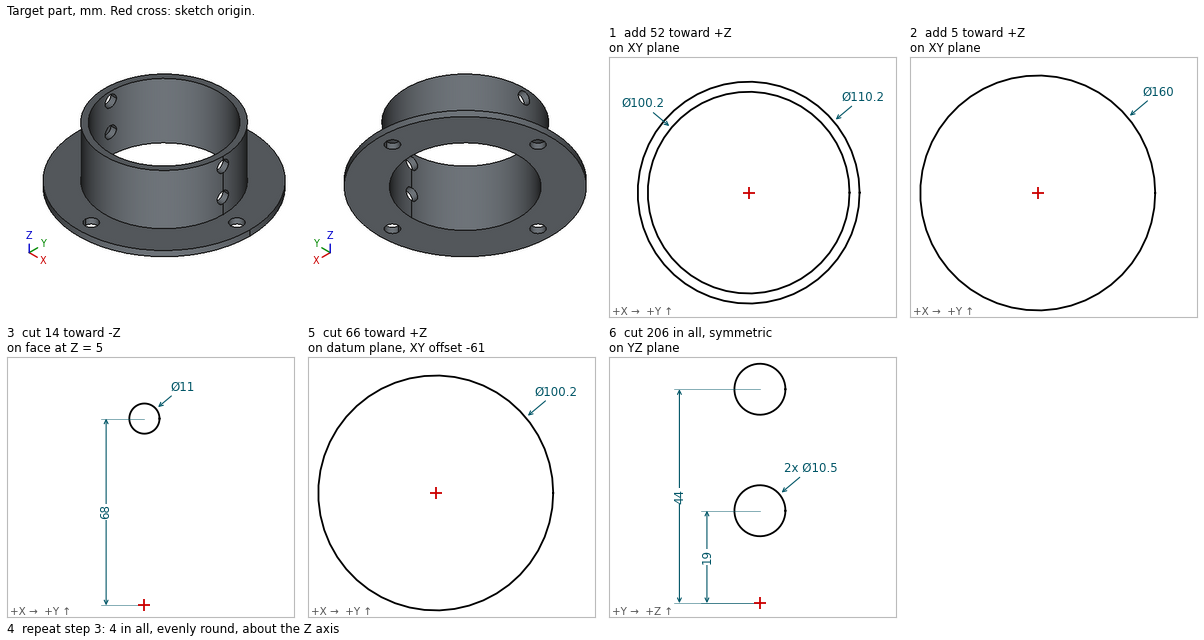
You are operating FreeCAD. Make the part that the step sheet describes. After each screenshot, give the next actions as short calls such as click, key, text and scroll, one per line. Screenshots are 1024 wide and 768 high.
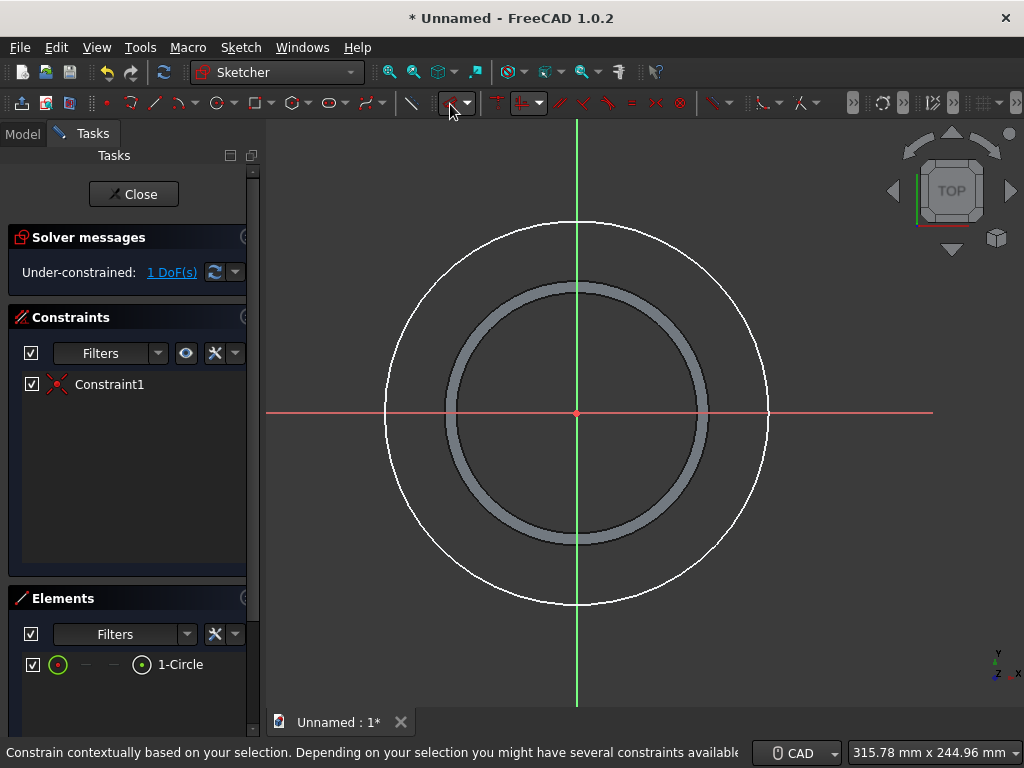
click(712, 277)
click(735, 254)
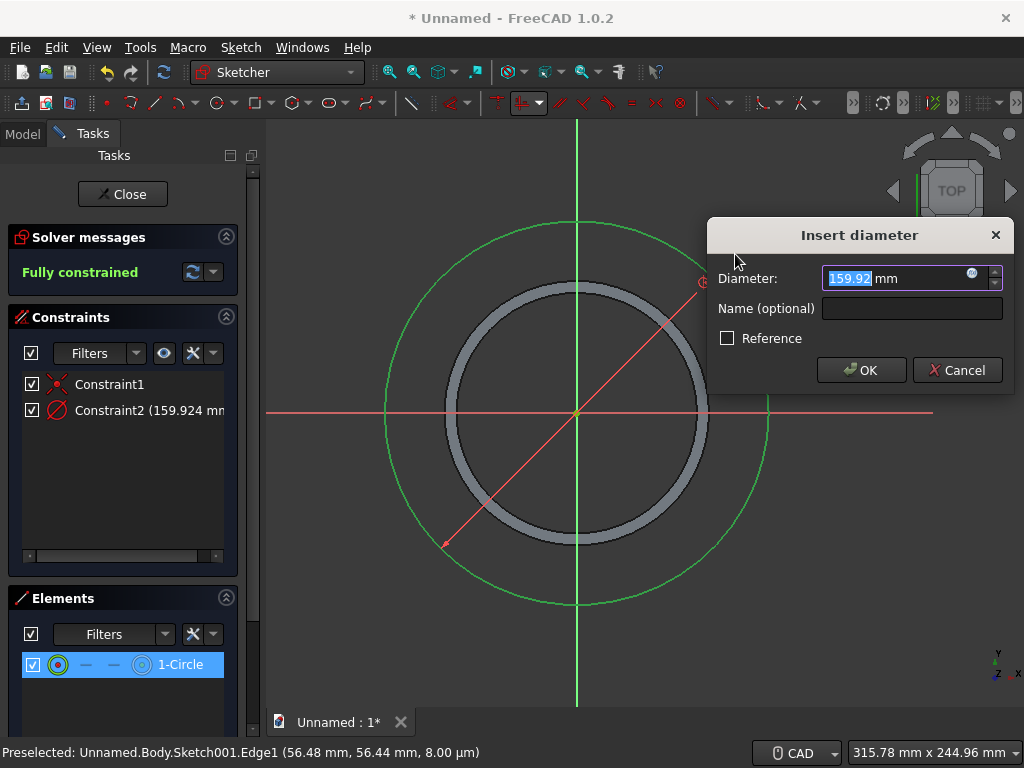
text(160)
key(Return)
key(Escape)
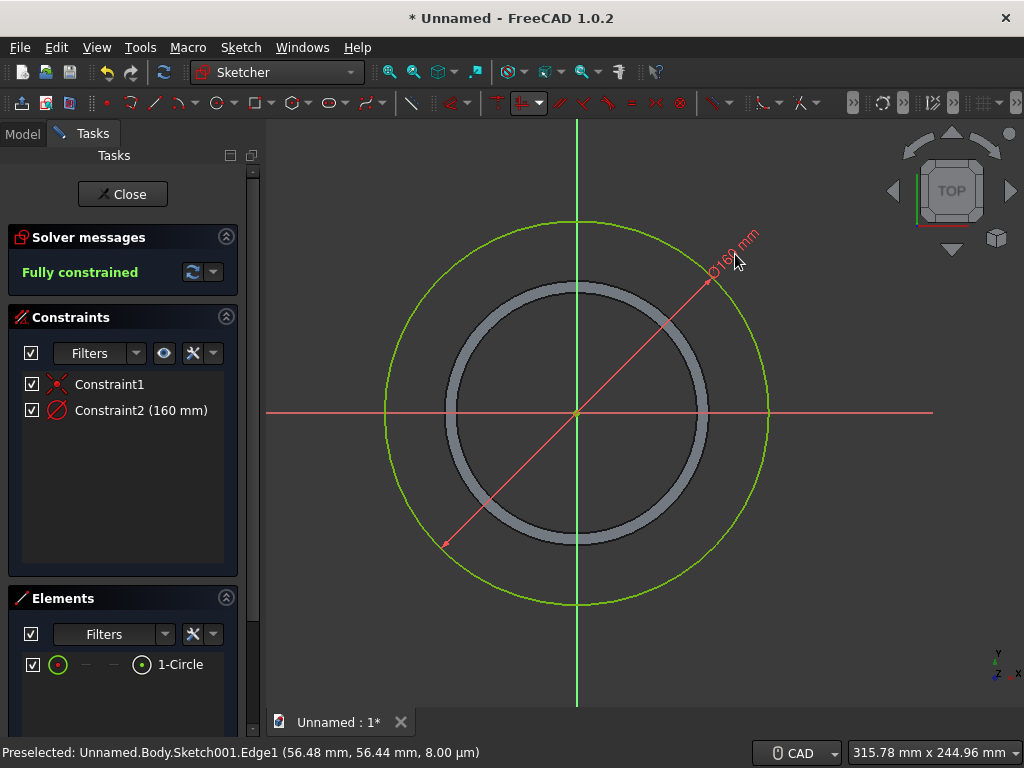
click(123, 194)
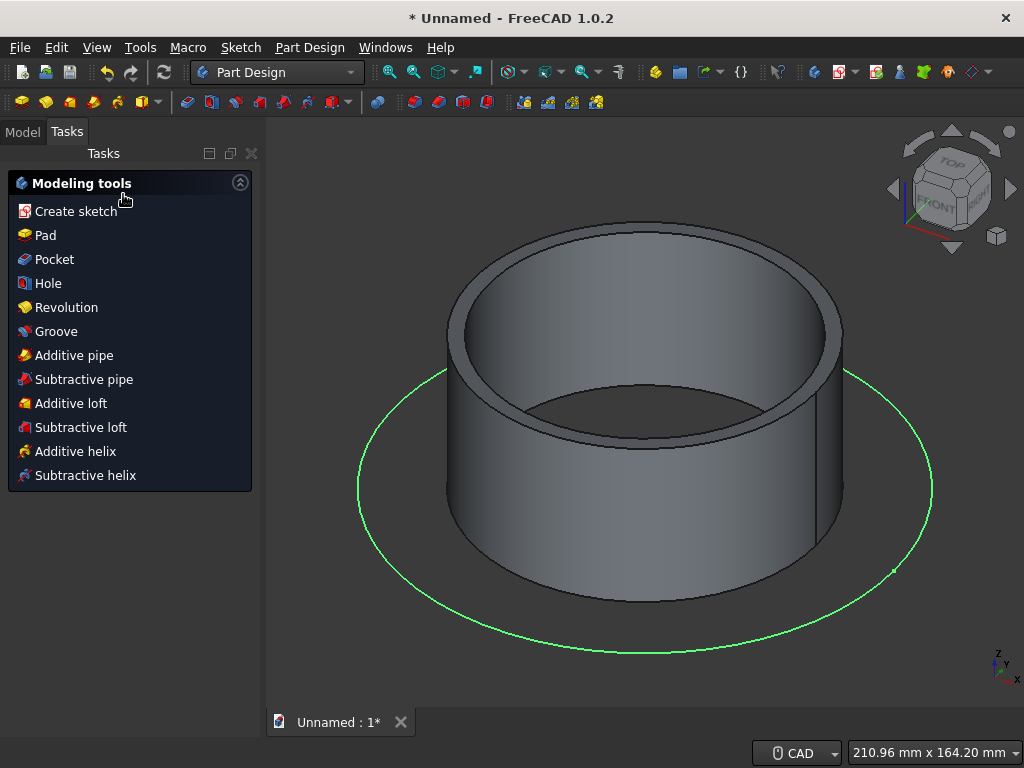
click(22, 102)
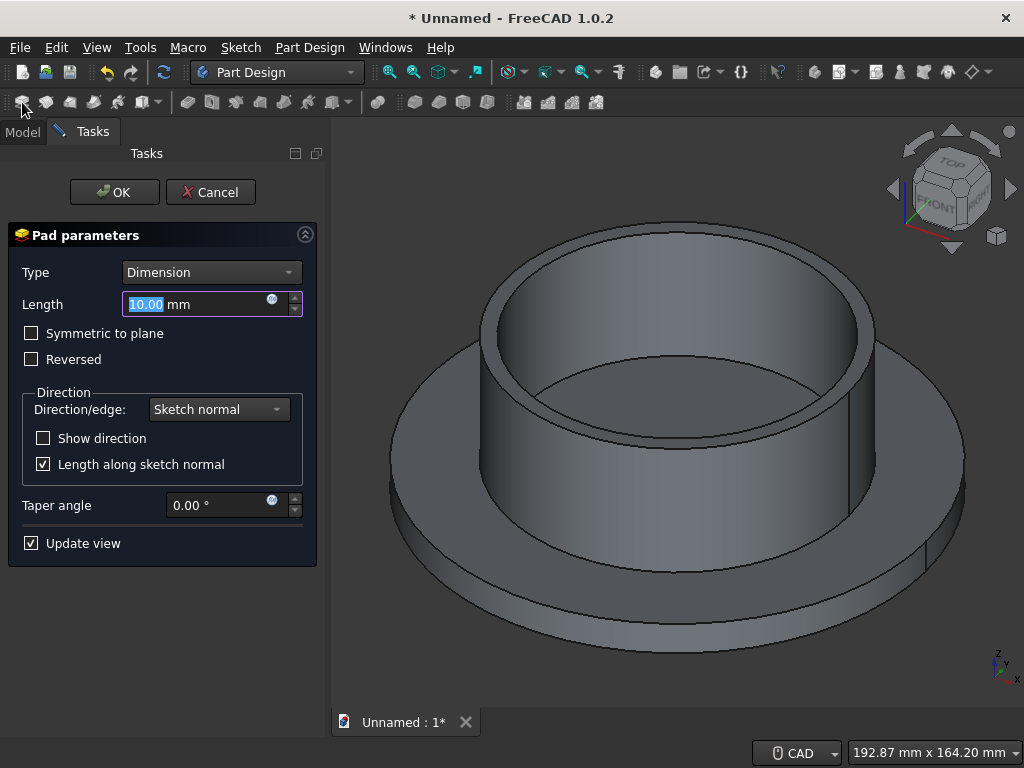
text(5)
key(Tab)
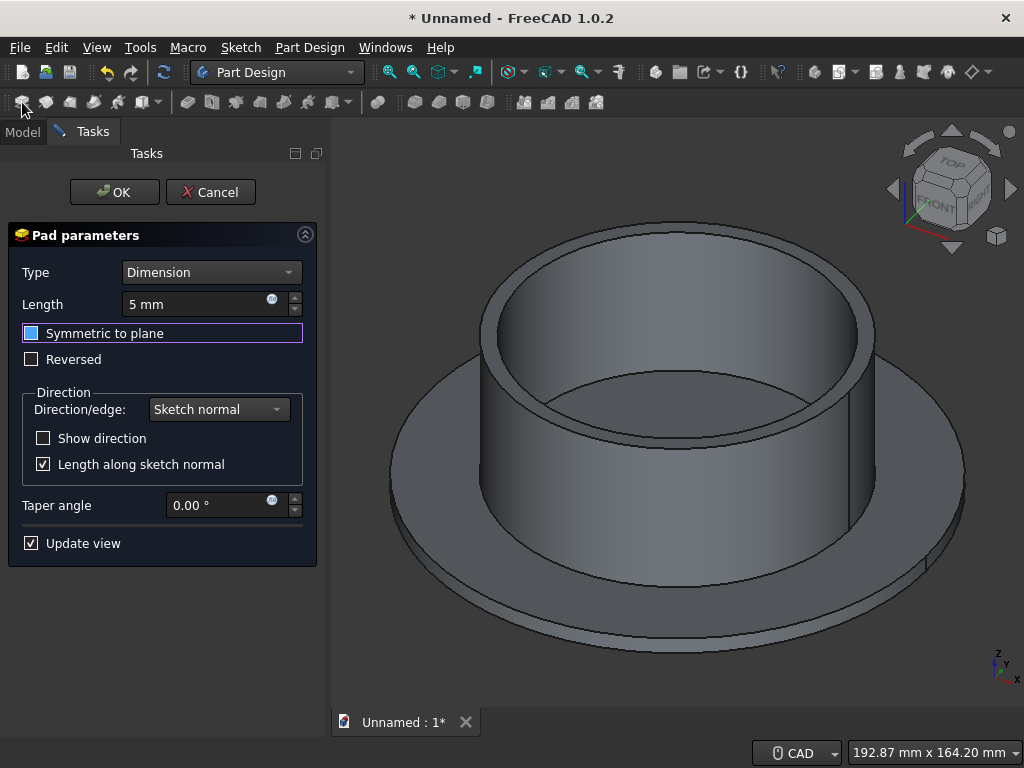
click(115, 192)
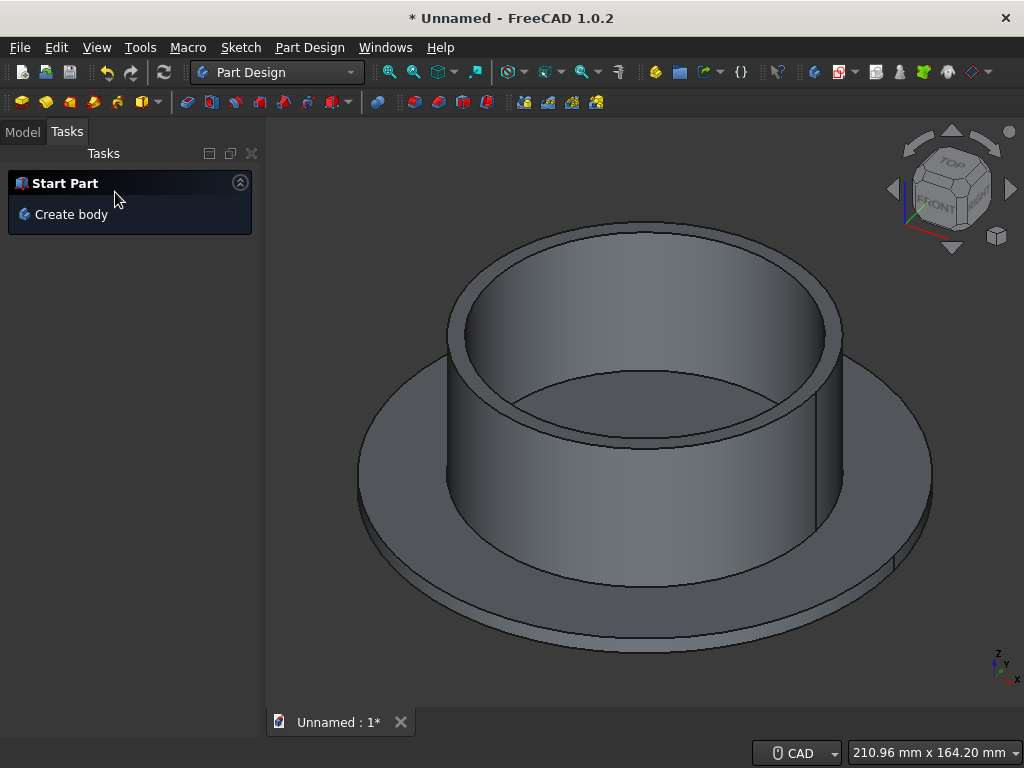
click(390, 72)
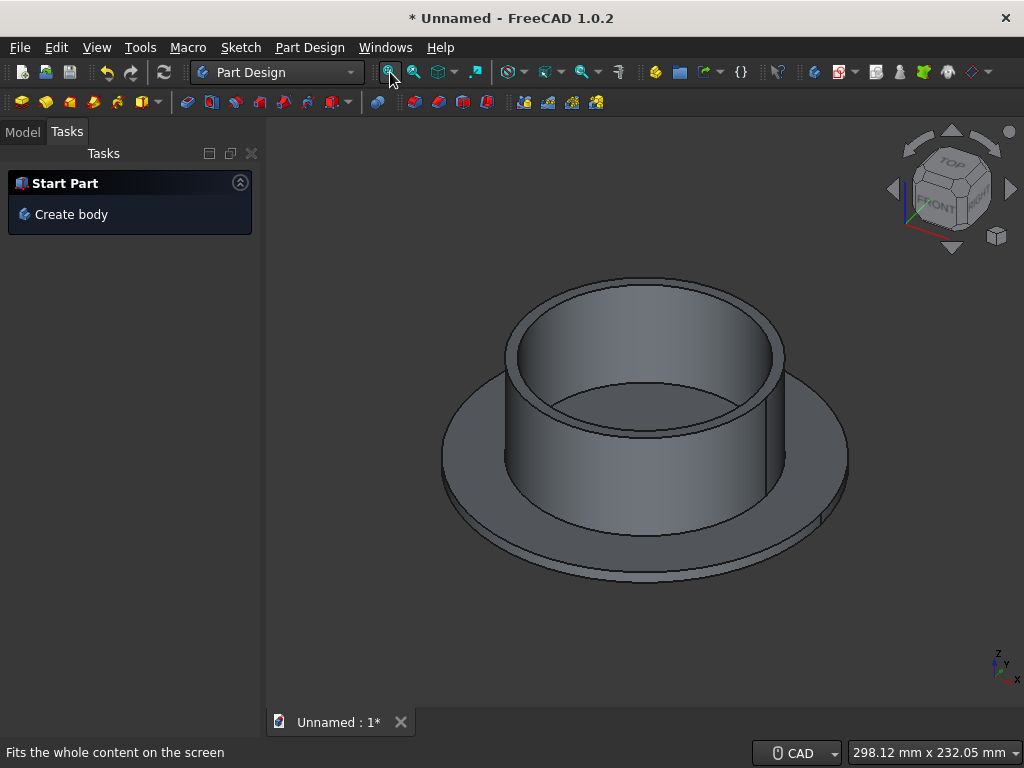
click(558, 541)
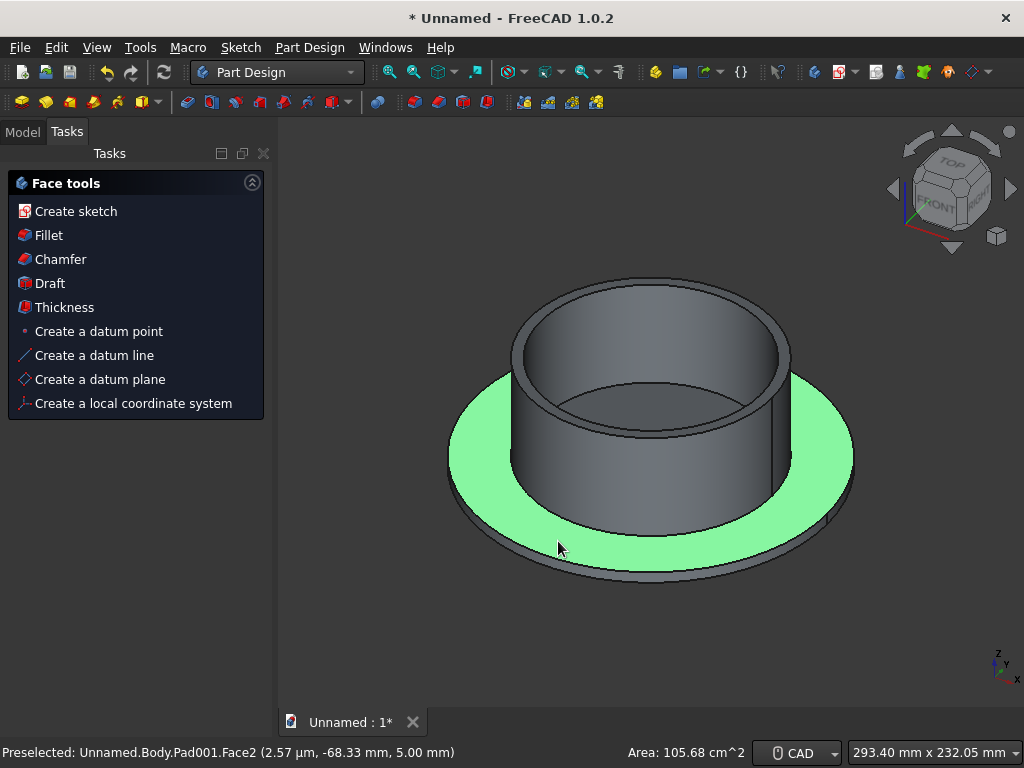
click(840, 72)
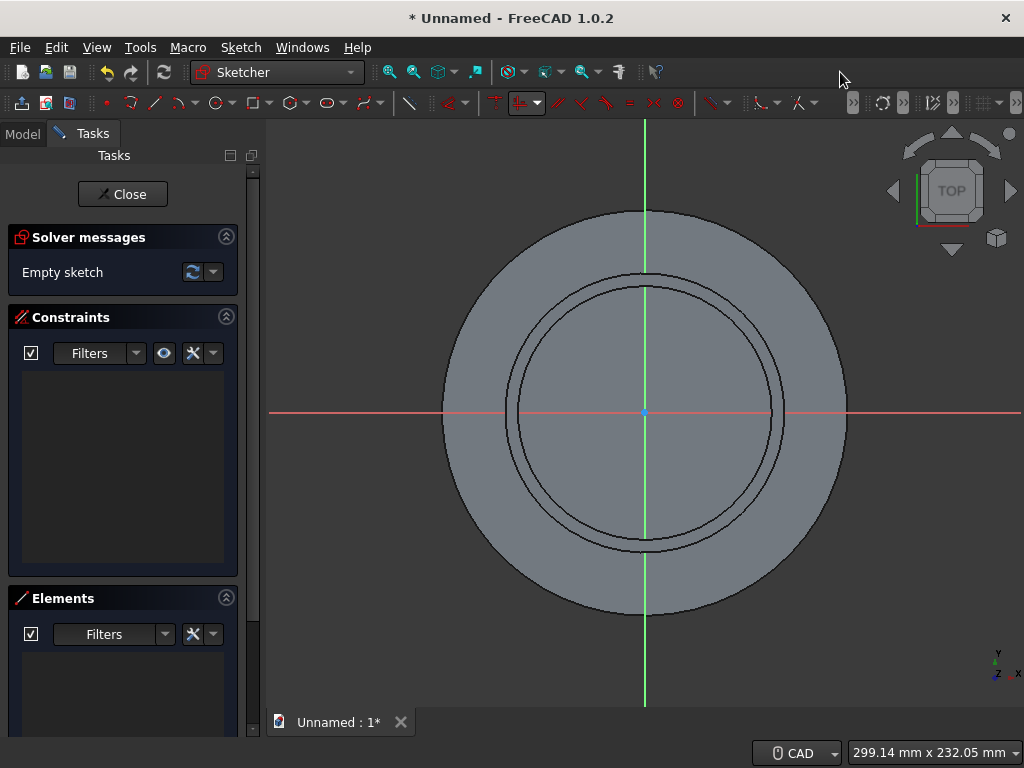
click(70, 104)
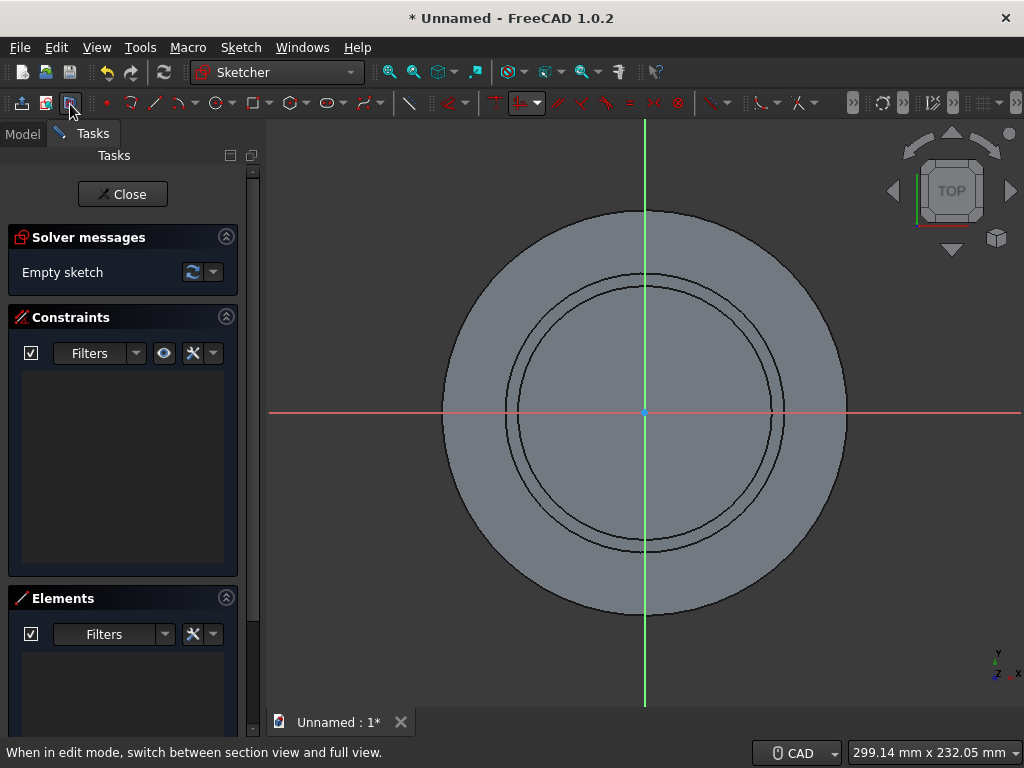
scroll(650, 227, up, 13)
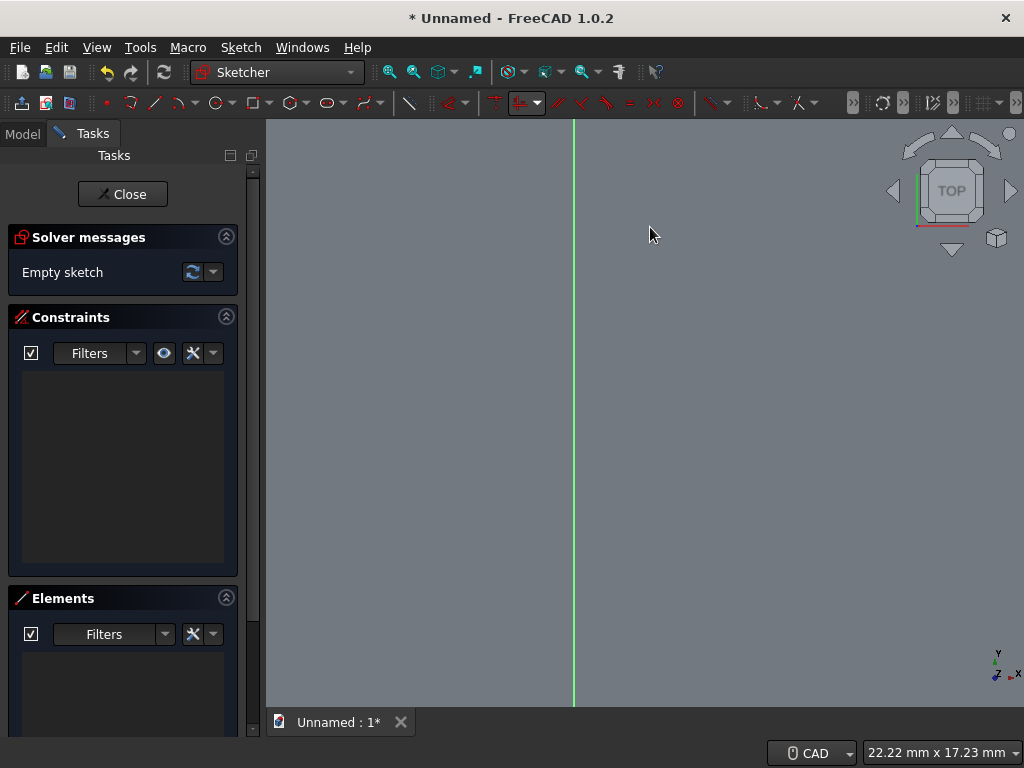
click(216, 104)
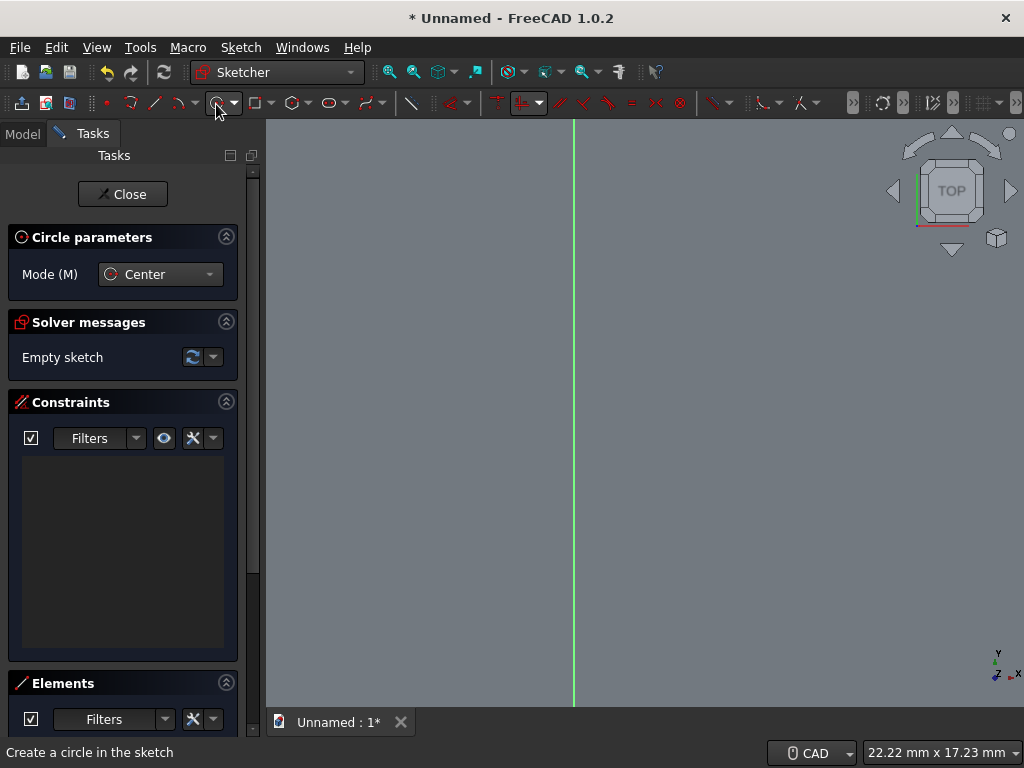
click(574, 409)
click(707, 276)
key(Escape)